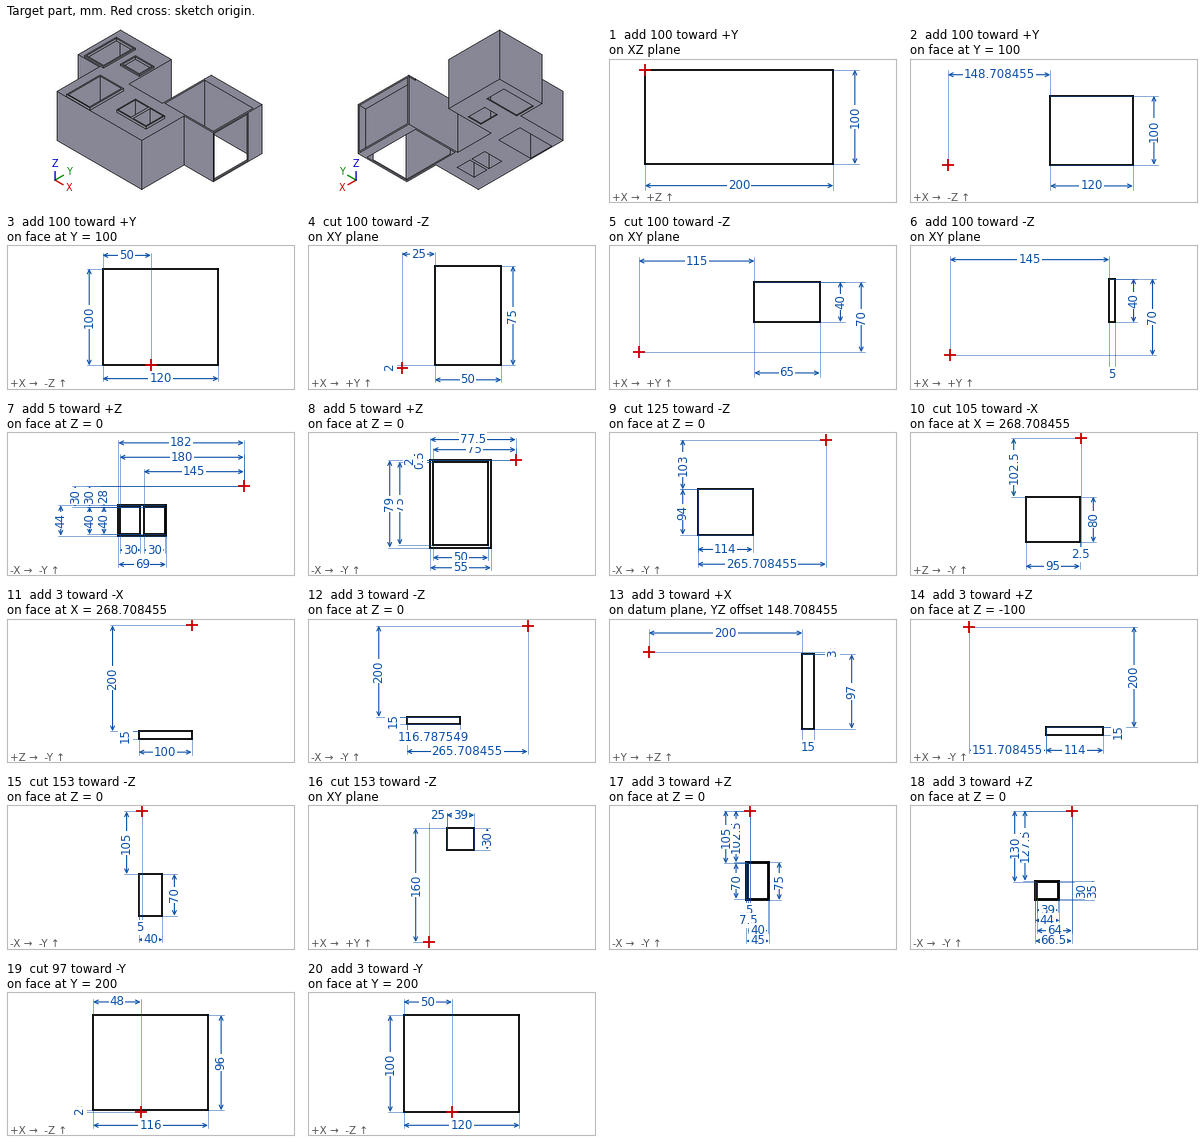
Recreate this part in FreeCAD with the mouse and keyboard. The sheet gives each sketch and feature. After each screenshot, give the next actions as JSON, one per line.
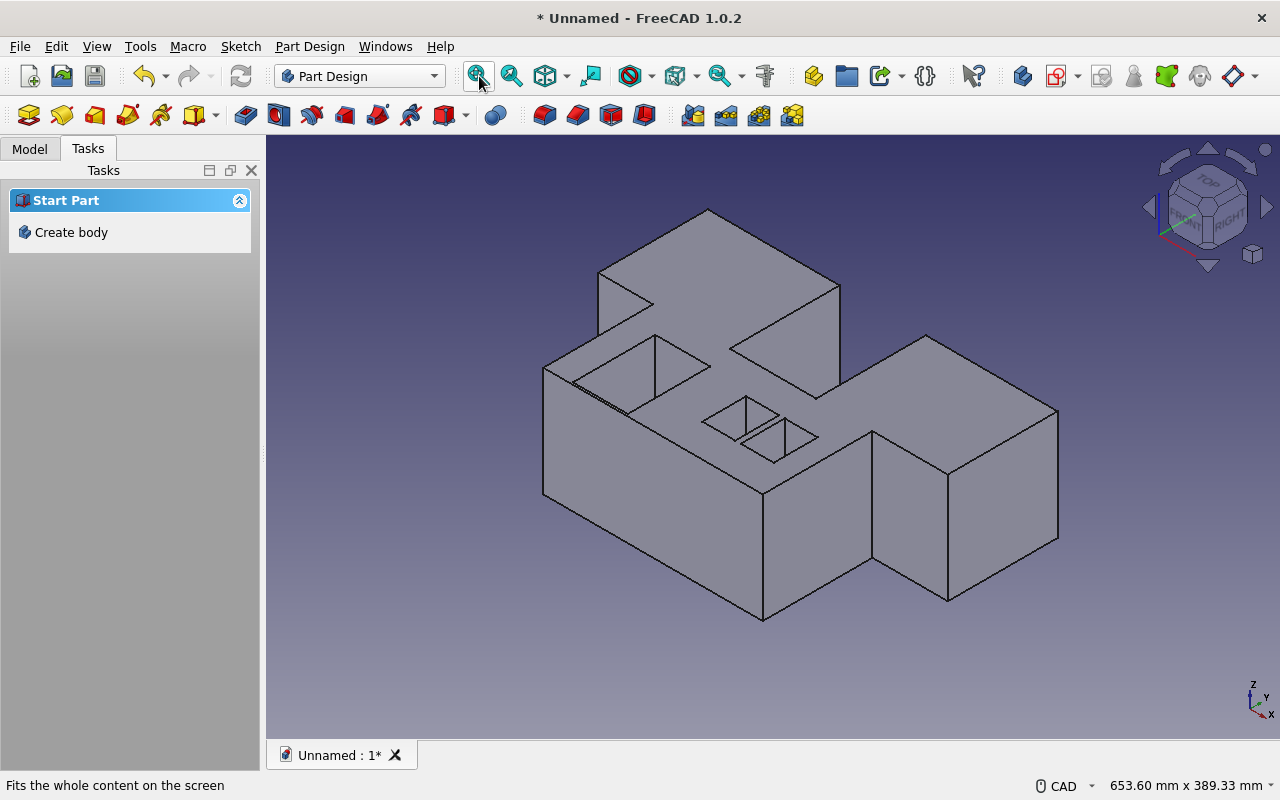
{"action": "left_click", "coordinate": [936, 394]}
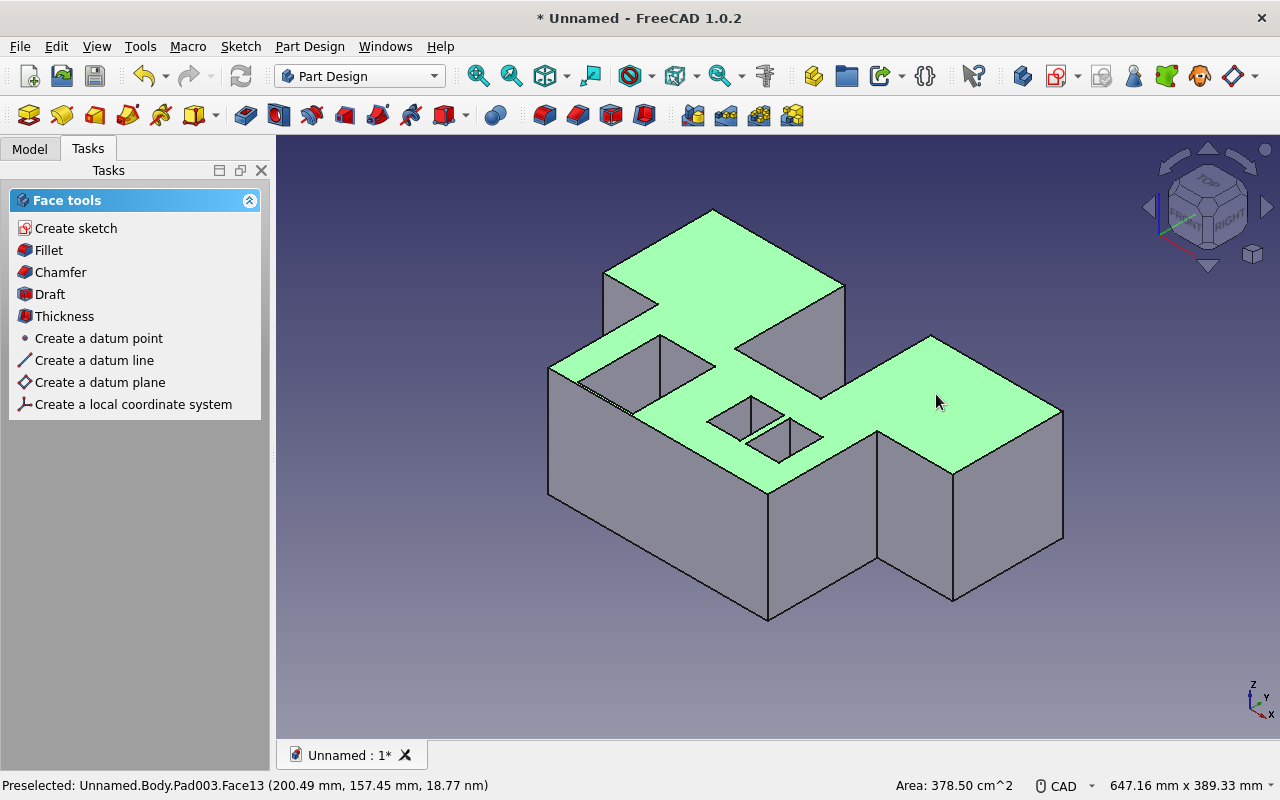
{"action": "left_click", "coordinate": [1056, 76]}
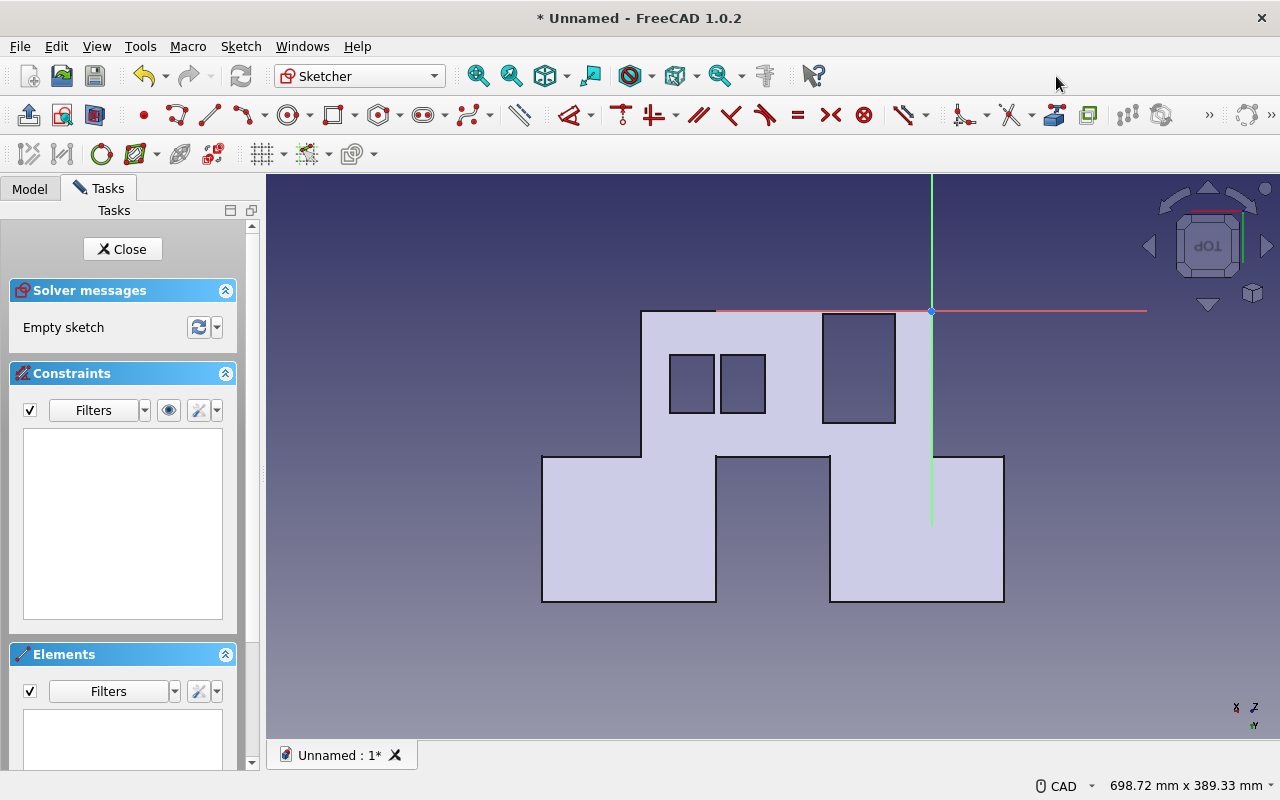
{"action": "scroll", "coordinate": [720, 370], "scroll_direction": "up", "scroll_amount": 9}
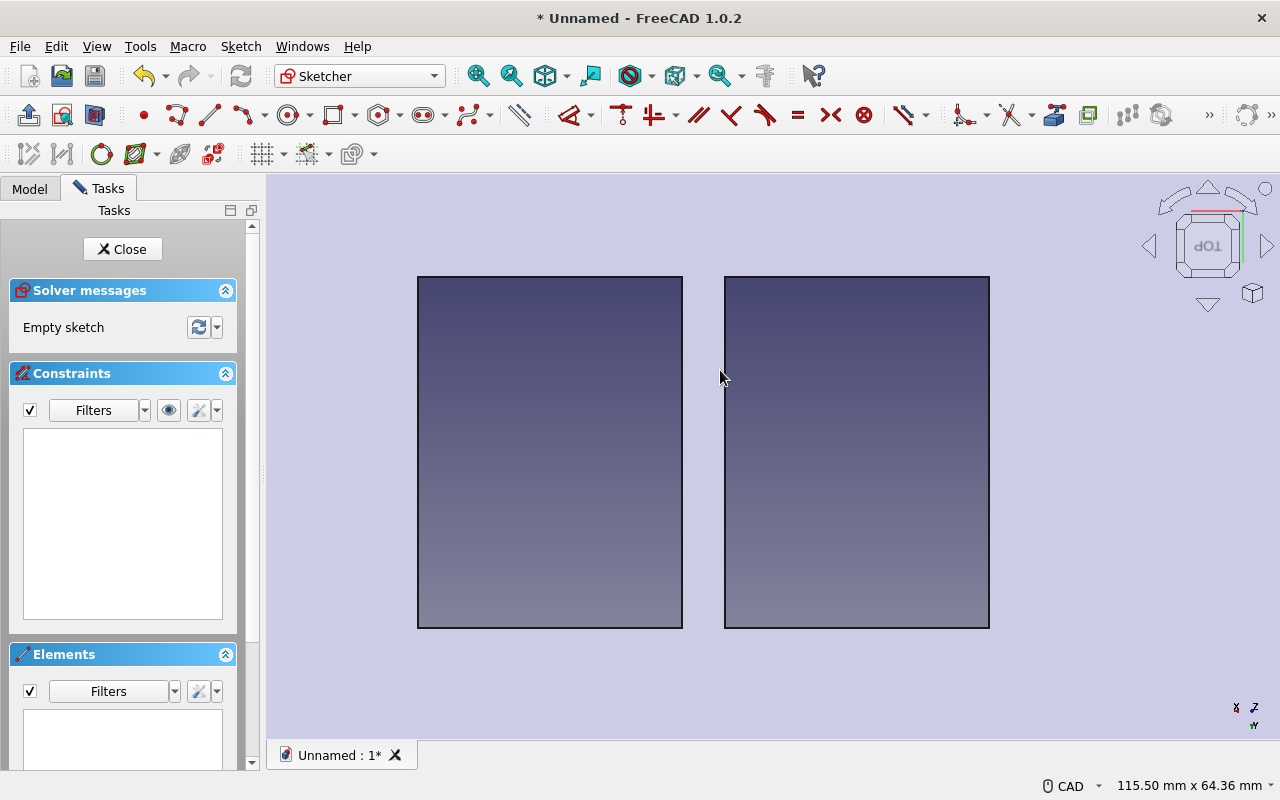
{"action": "left_click", "coordinate": [332, 116]}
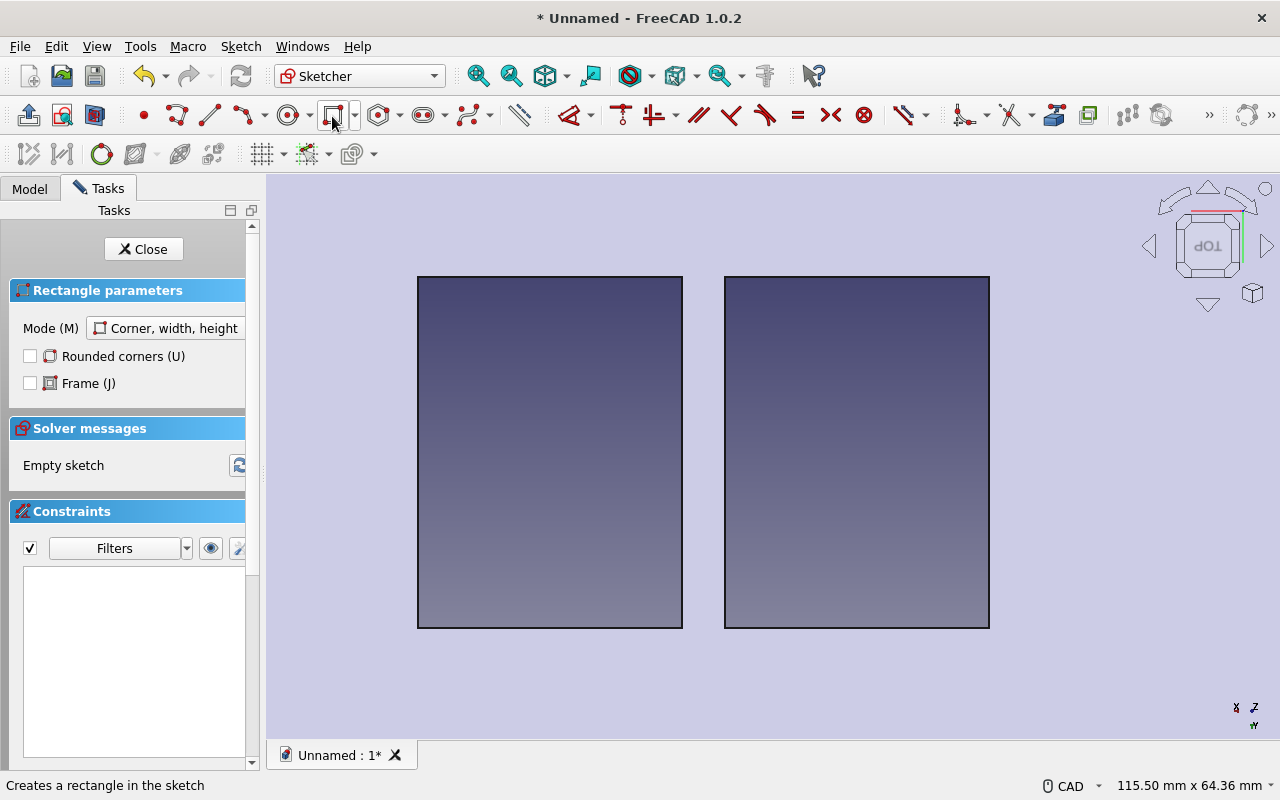
{"action": "left_click", "coordinate": [401, 259]}
{"action": "mouse_move", "coordinate": [1006, 646]}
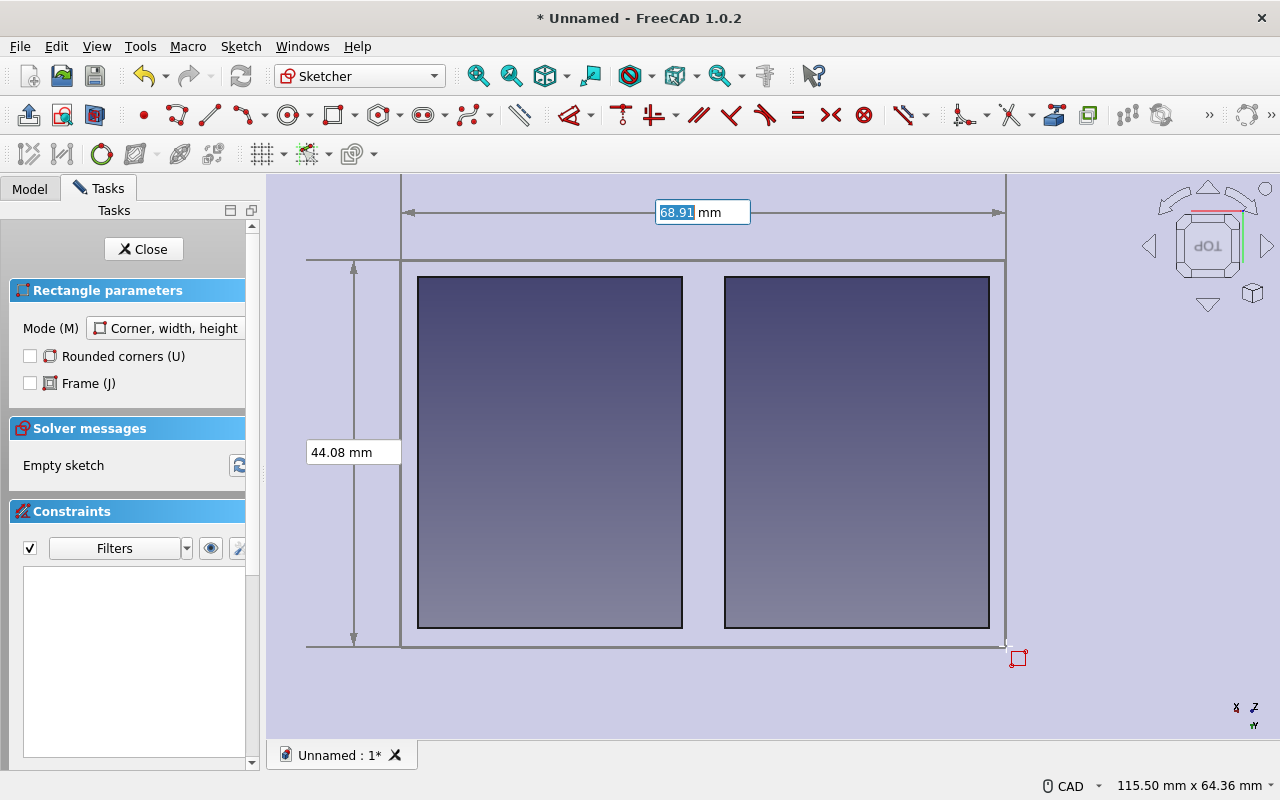
{"action": "type", "text": "69"}
{"action": "key", "text": "Tab"}
{"action": "type", "text": "44"}
{"action": "key", "text": "Return"}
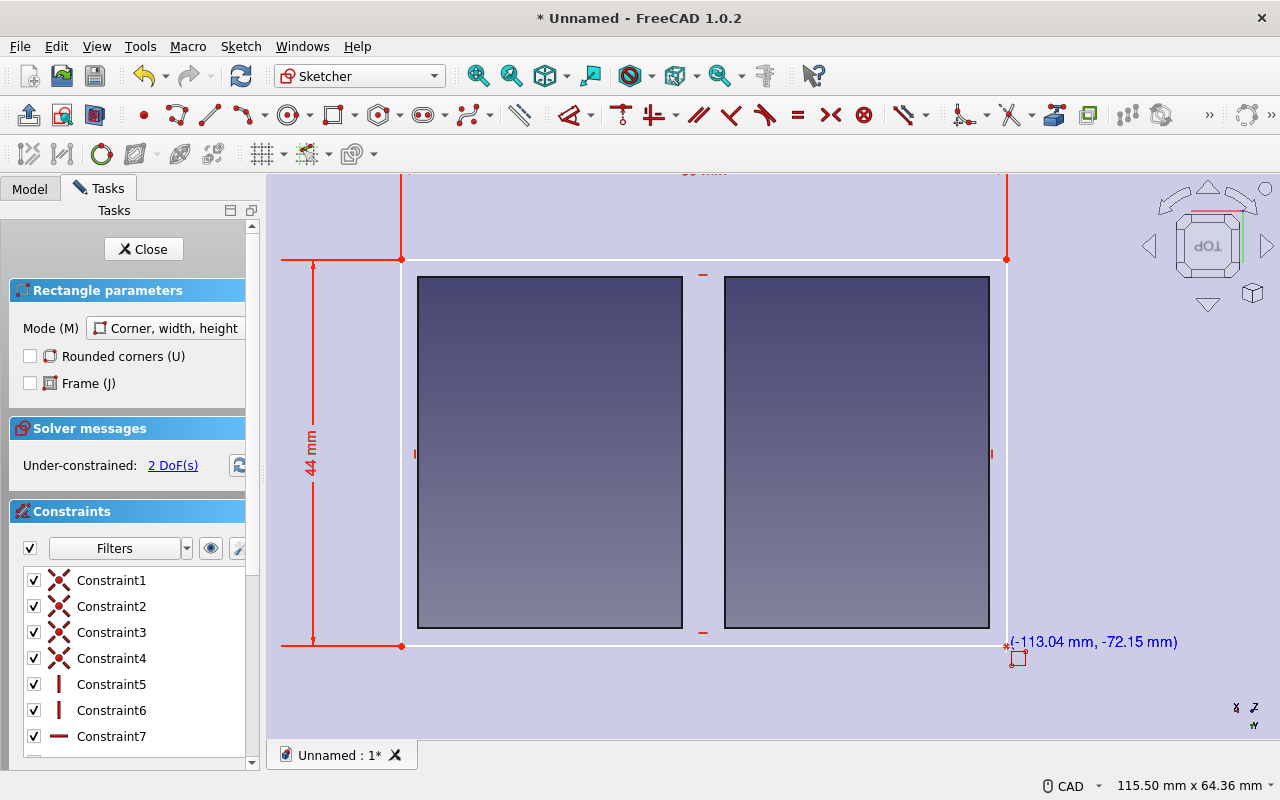
{"action": "left_click", "coordinate": [725, 277]}
{"action": "mouse_move", "coordinate": [989, 628]}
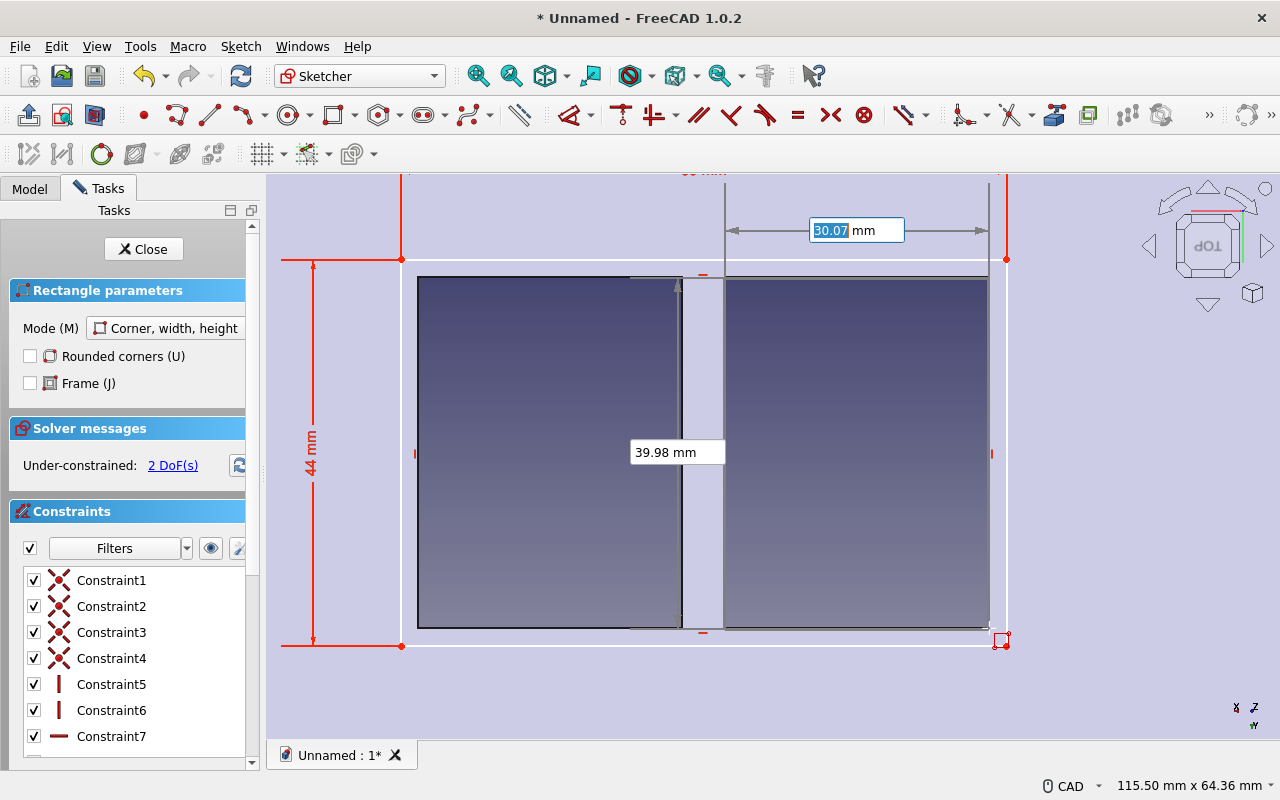
{"action": "type", "text": "30"}
{"action": "key", "text": "Tab"}
{"action": "type", "text": "40"}
{"action": "key", "text": "Return"}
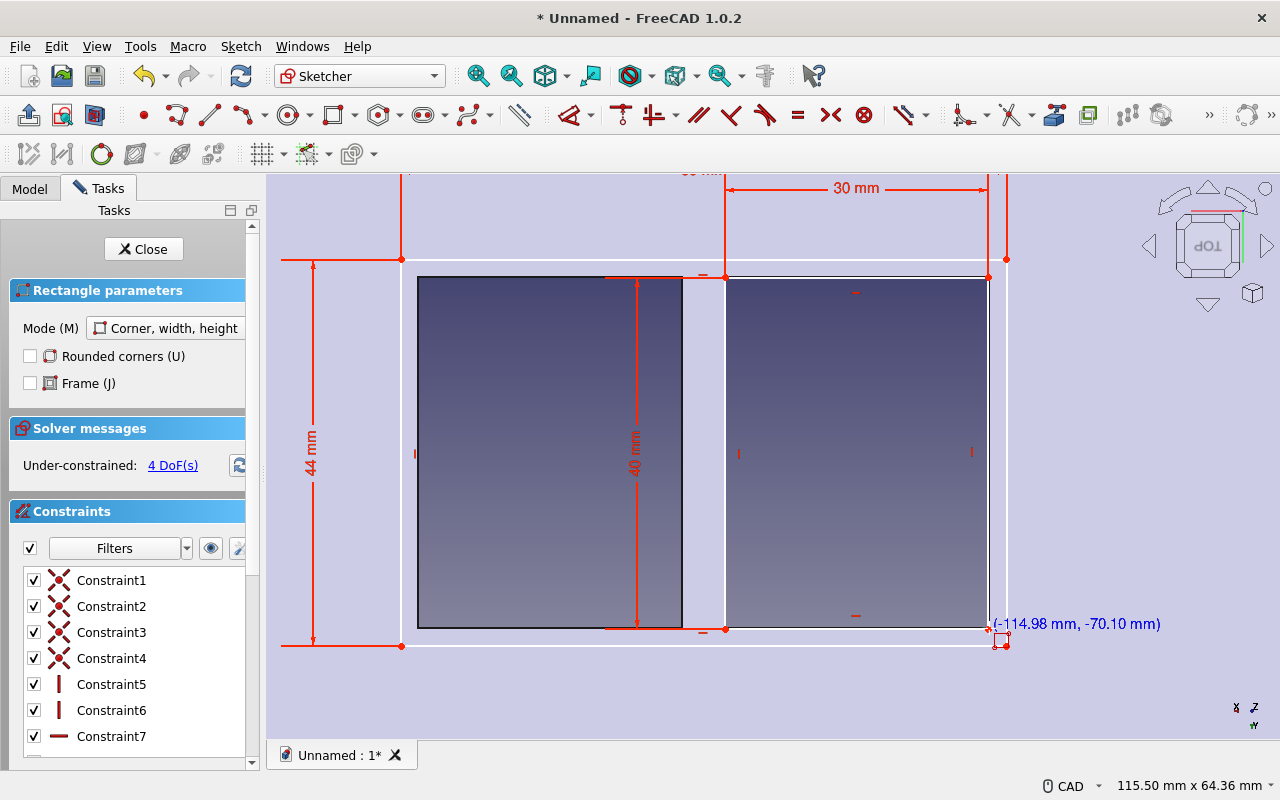
{"action": "left_click", "coordinate": [418, 277]}
{"action": "mouse_move", "coordinate": [682, 628]}